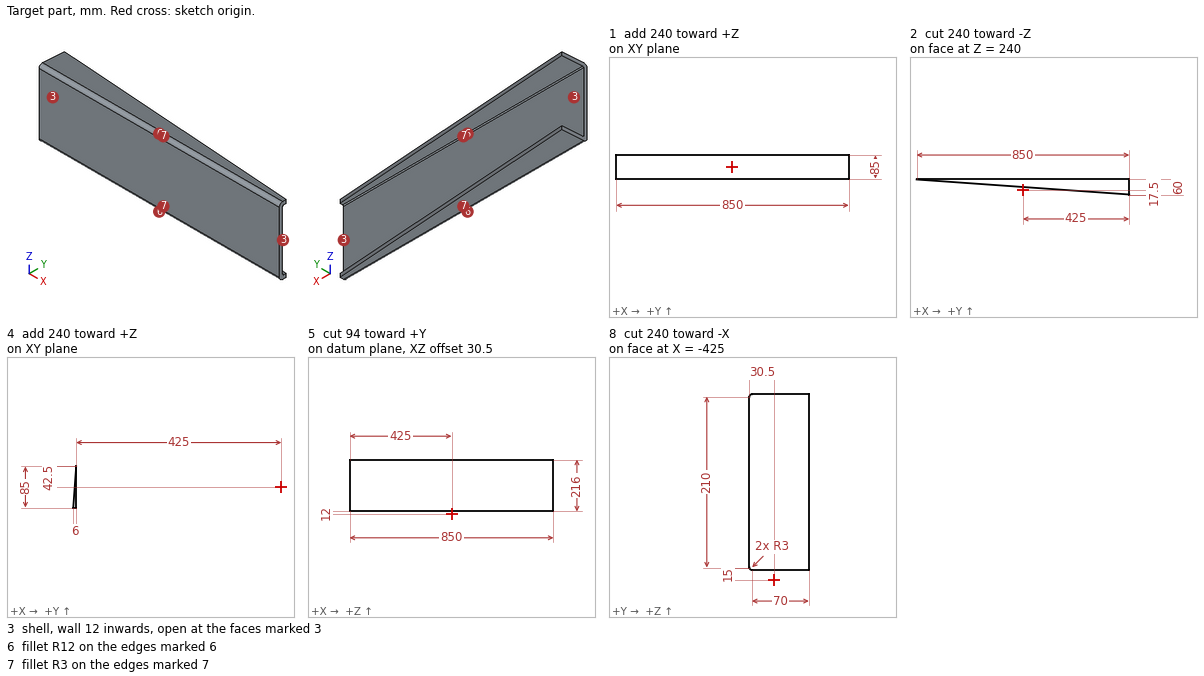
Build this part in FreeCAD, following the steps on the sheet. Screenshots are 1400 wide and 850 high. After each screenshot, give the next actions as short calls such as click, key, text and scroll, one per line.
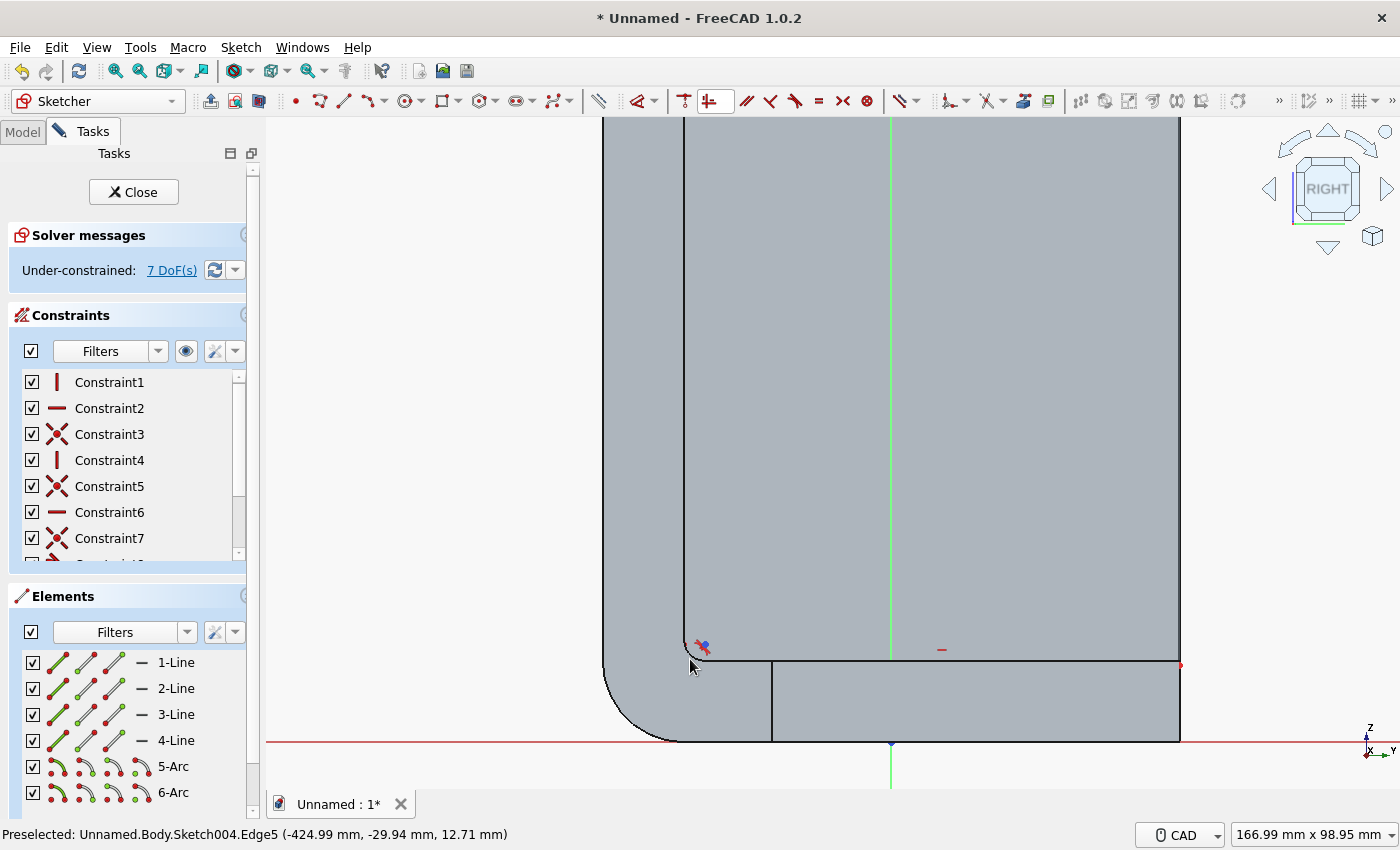
scroll(692, 662, down, 6)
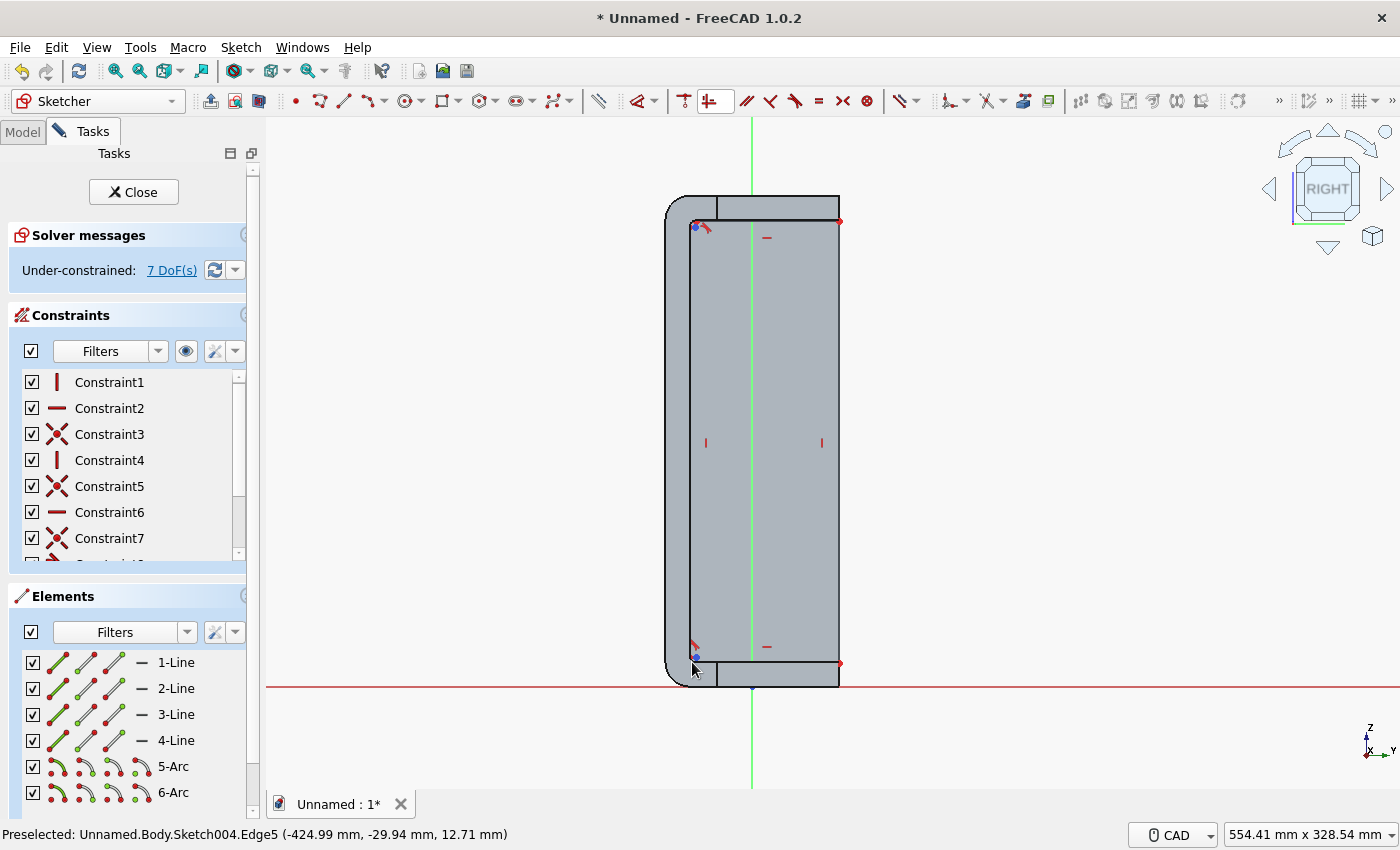
click(796, 221)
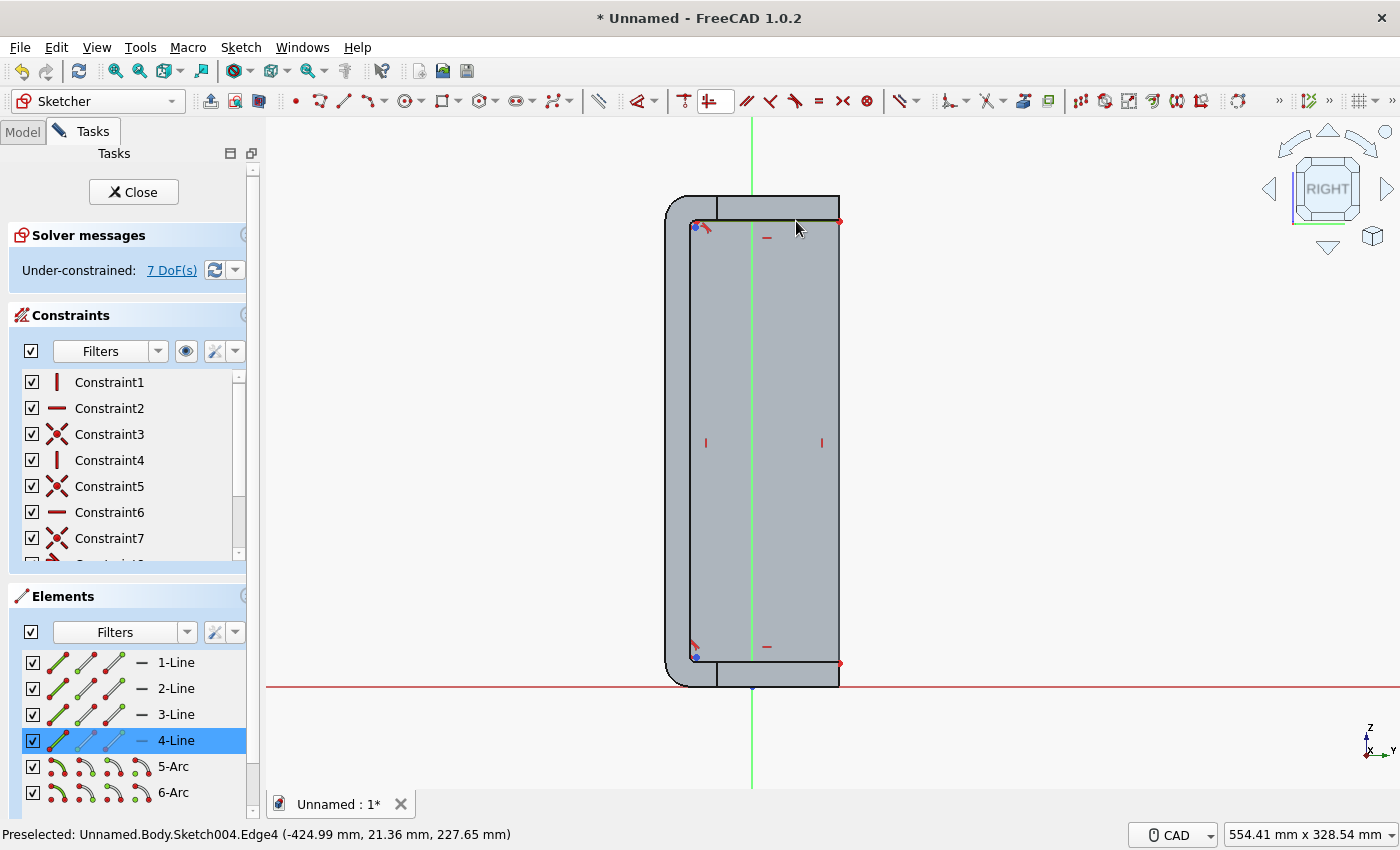
scroll(692, 223, up, 6)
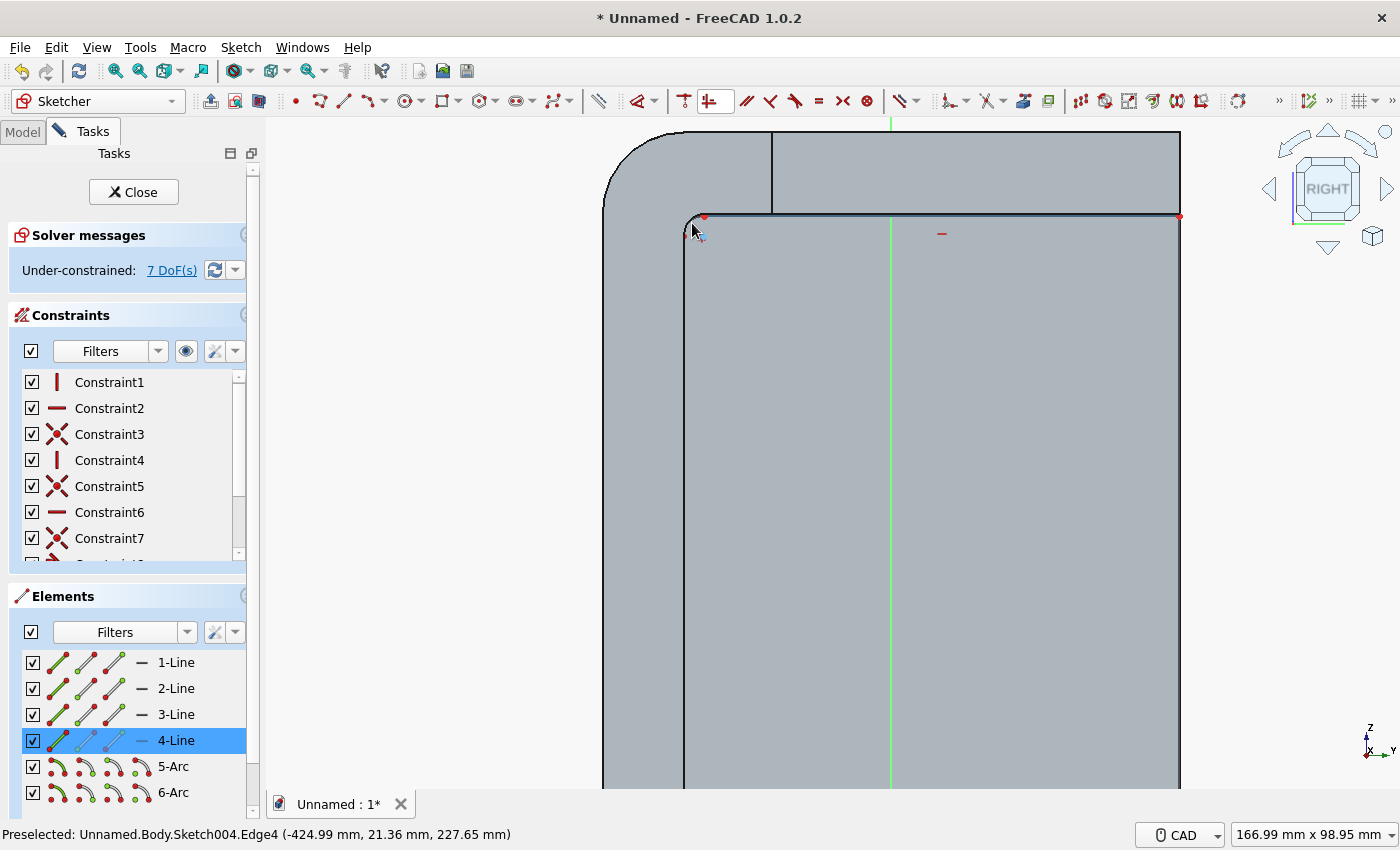
click(690, 222)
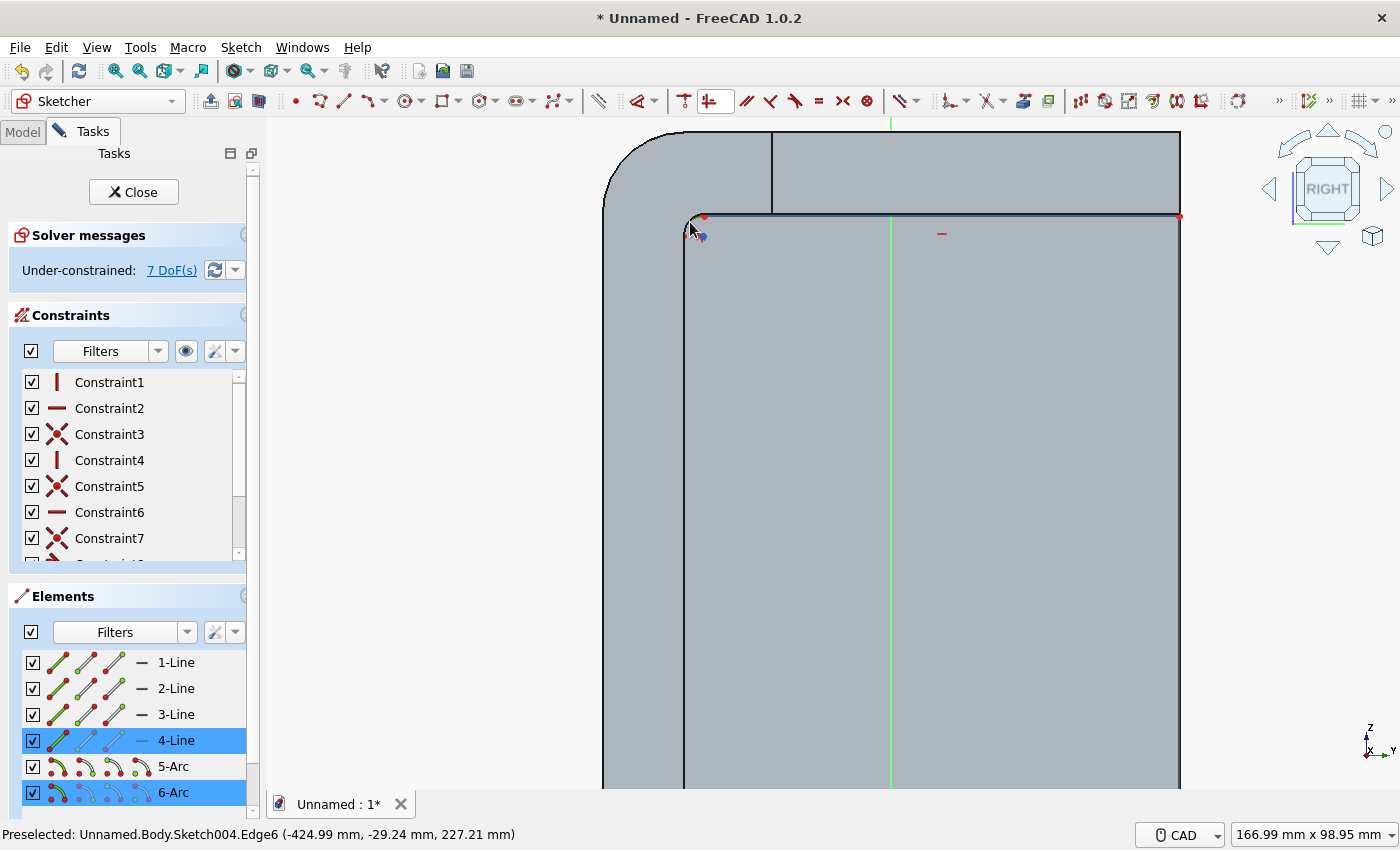
click(796, 102)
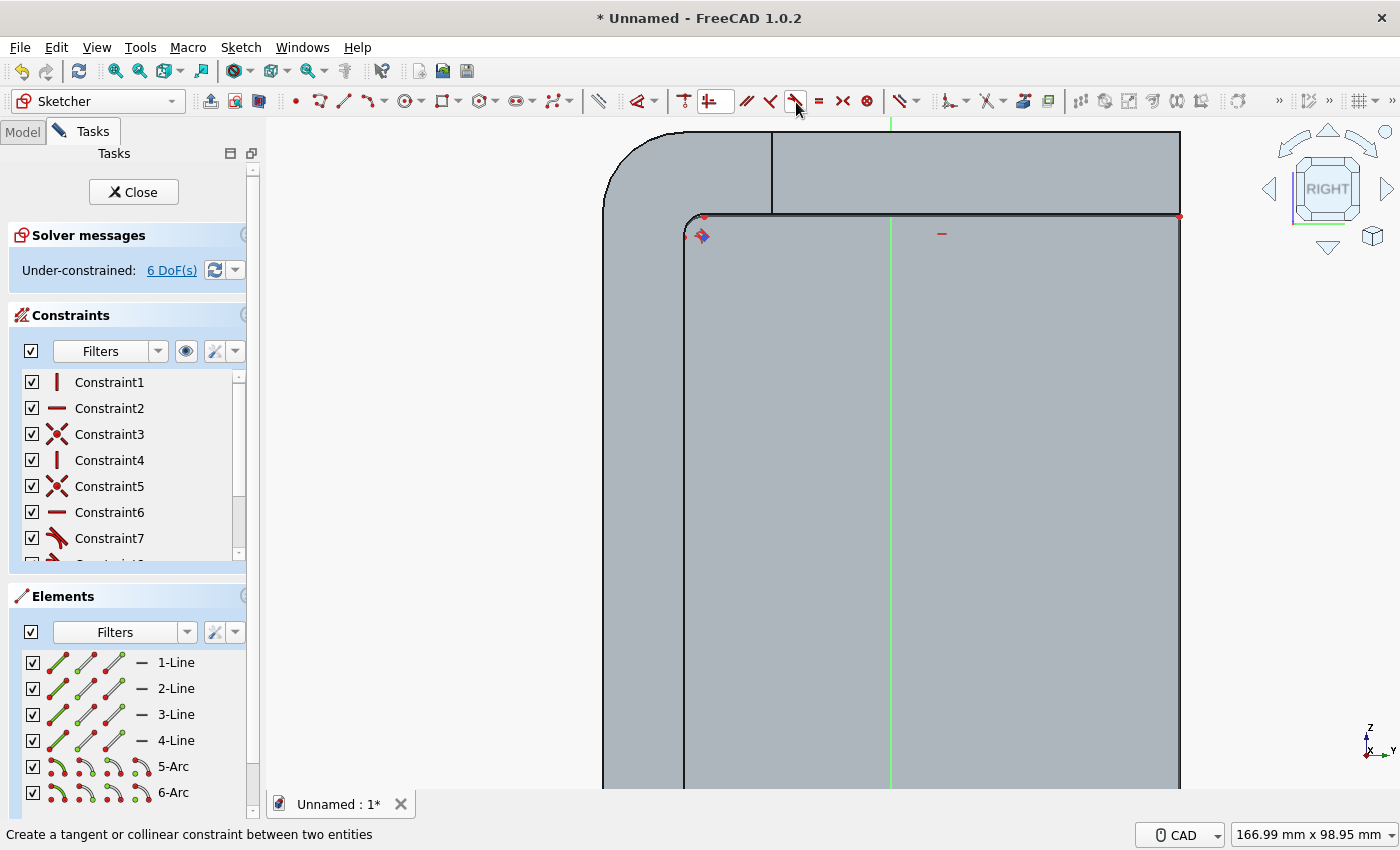
scroll(692, 222, down, 6)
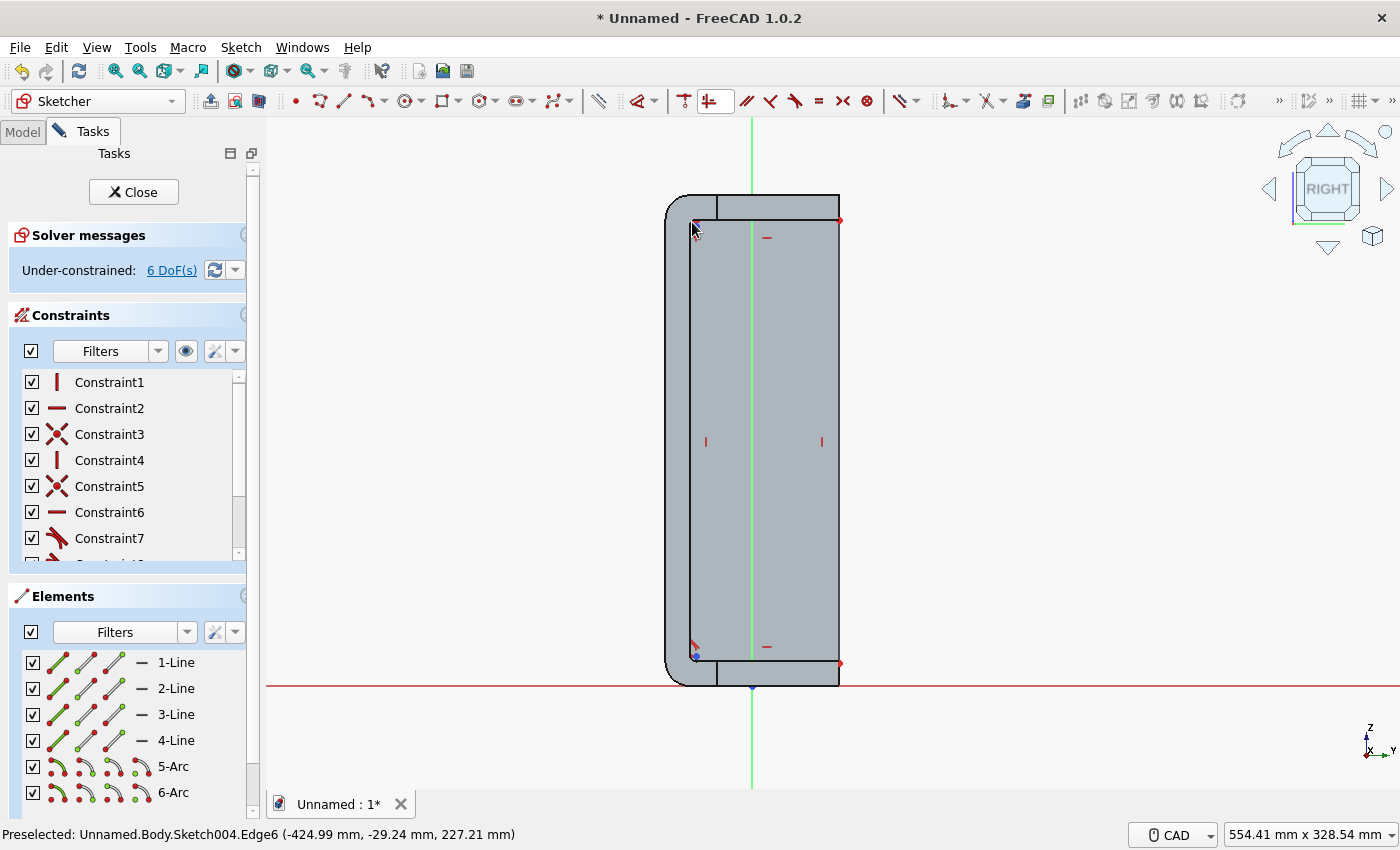
scroll(690, 659, up, 8)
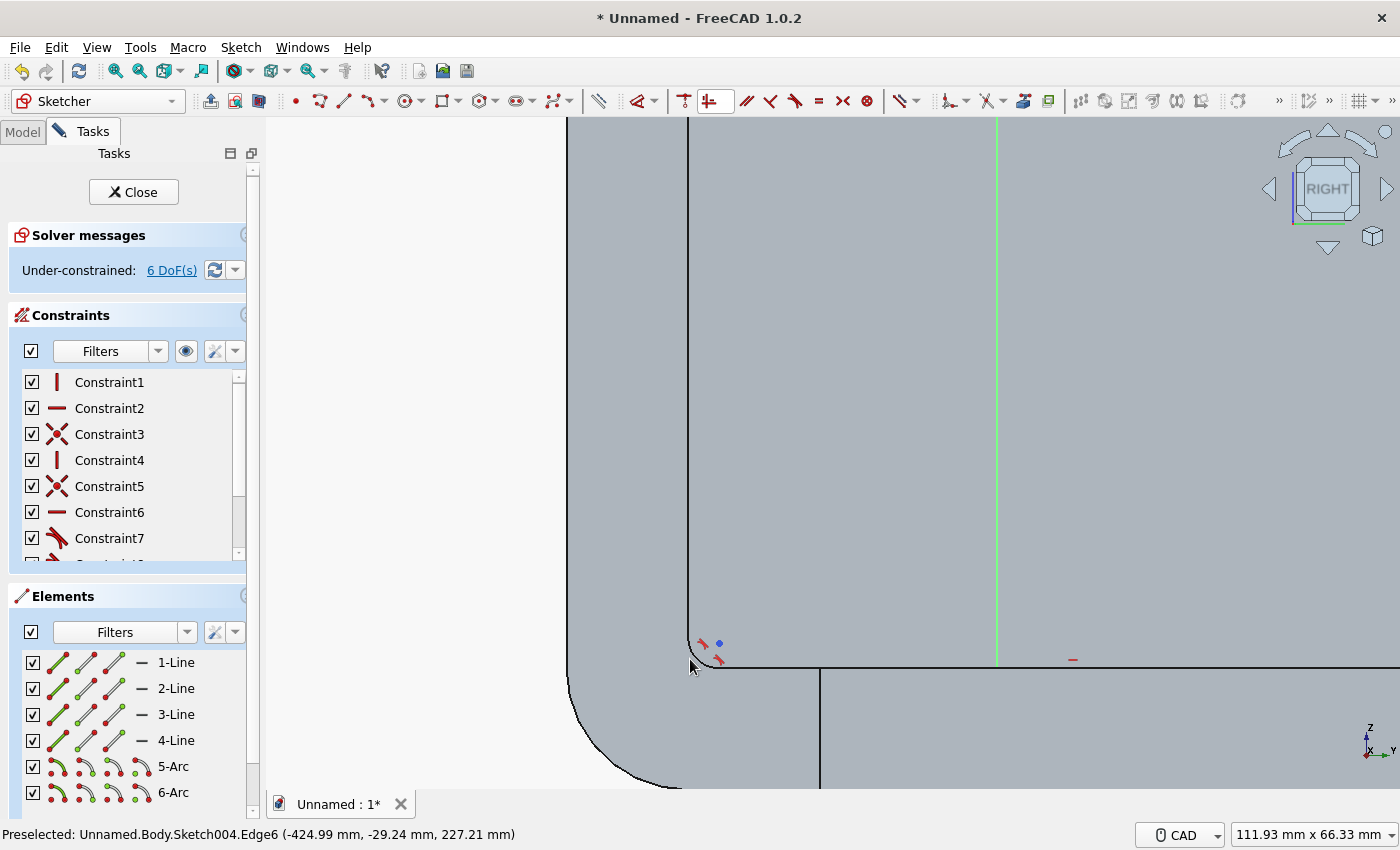
click(690, 658)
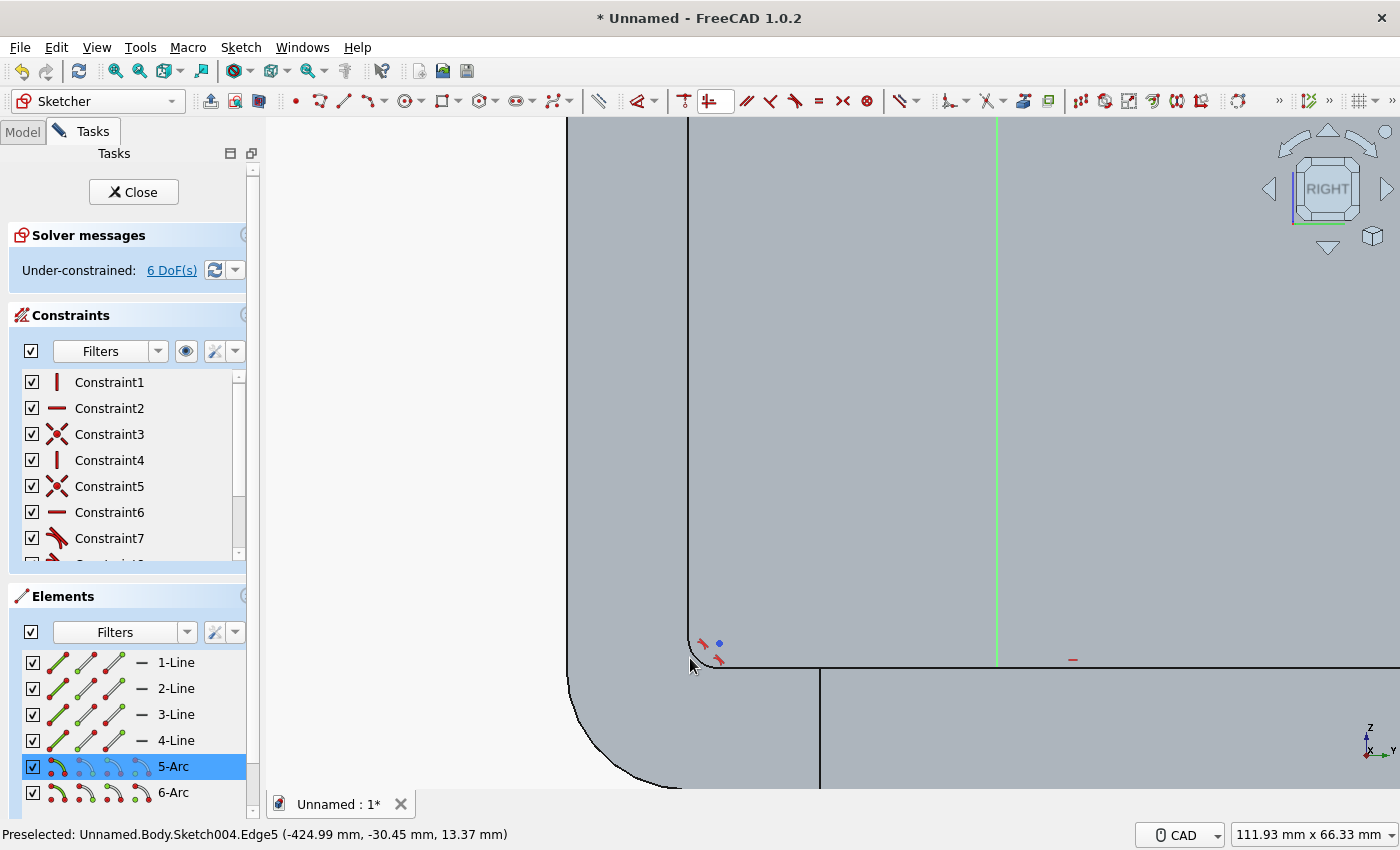
scroll(690, 660, down, 8)